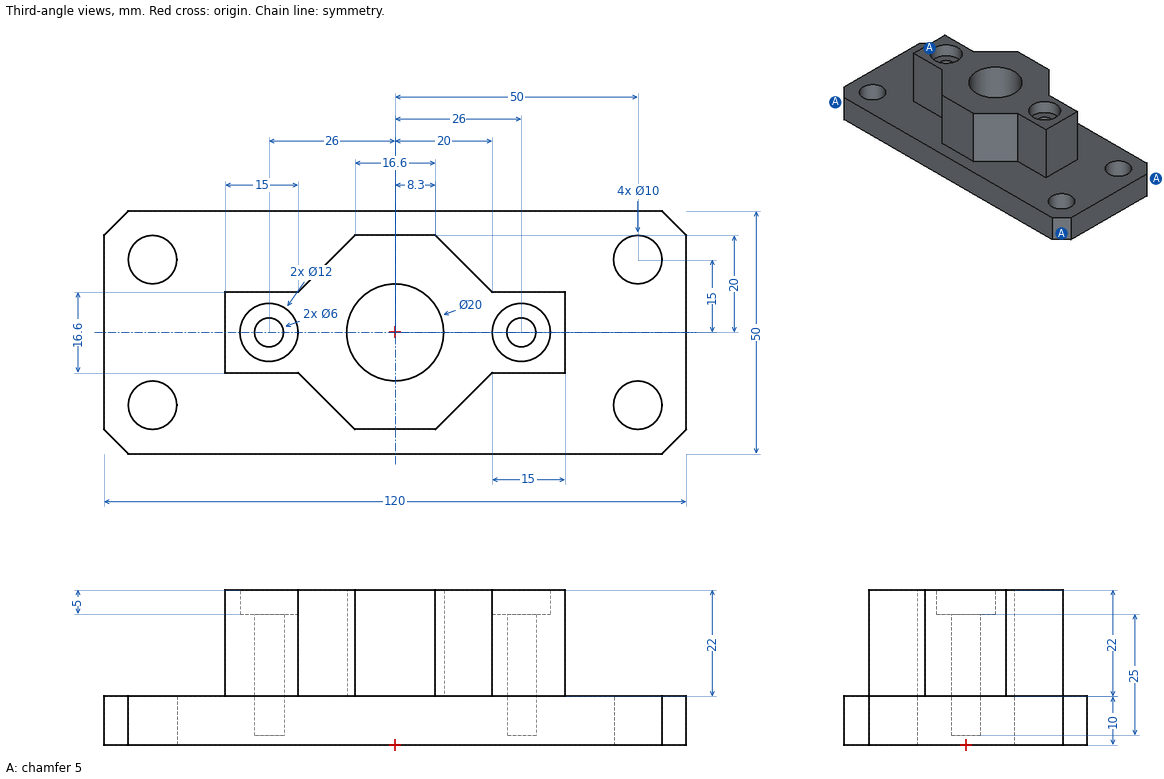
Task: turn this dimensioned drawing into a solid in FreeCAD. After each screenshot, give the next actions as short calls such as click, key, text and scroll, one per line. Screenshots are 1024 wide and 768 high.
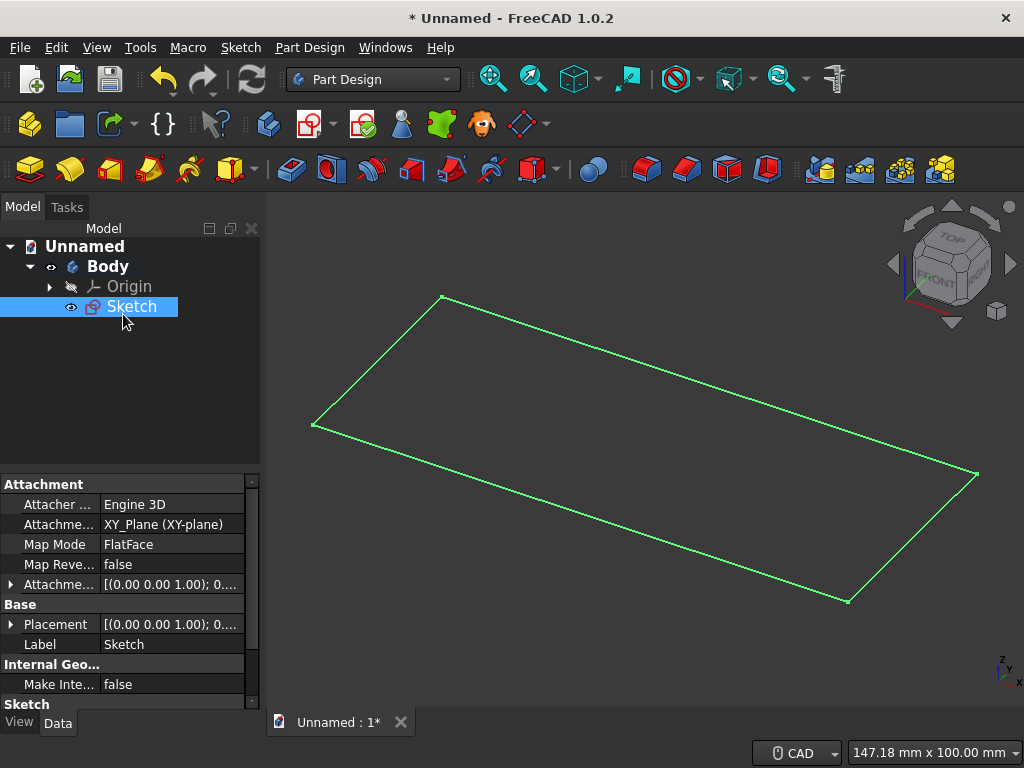
click(30, 170)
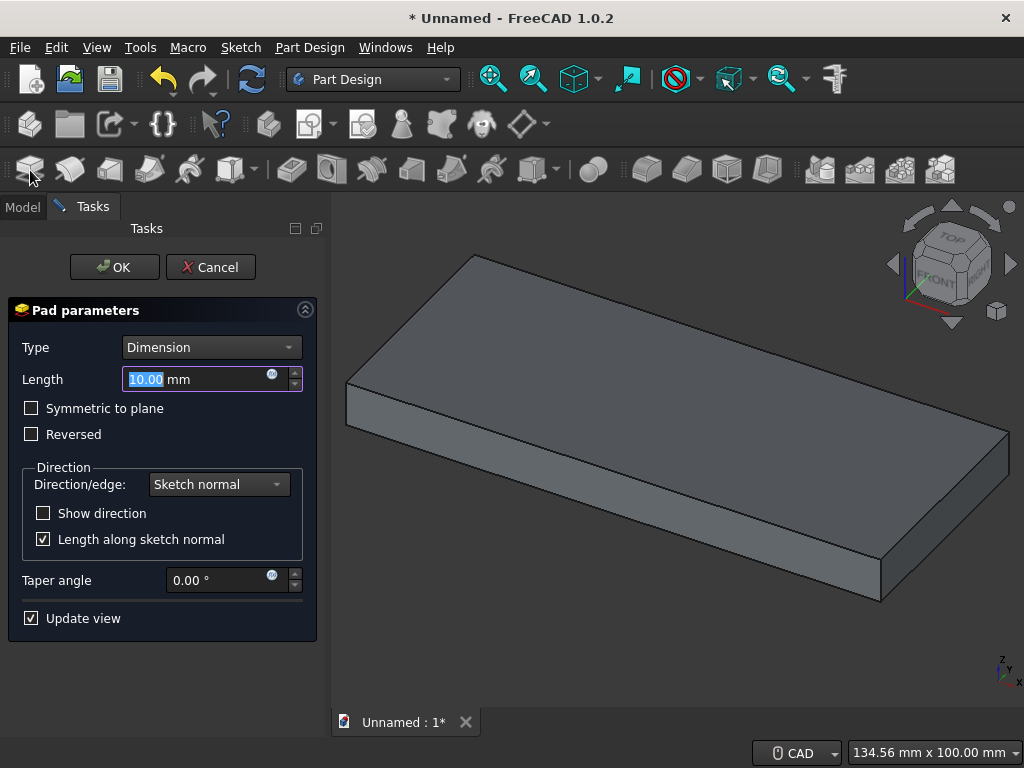
text(10)
key(Tab)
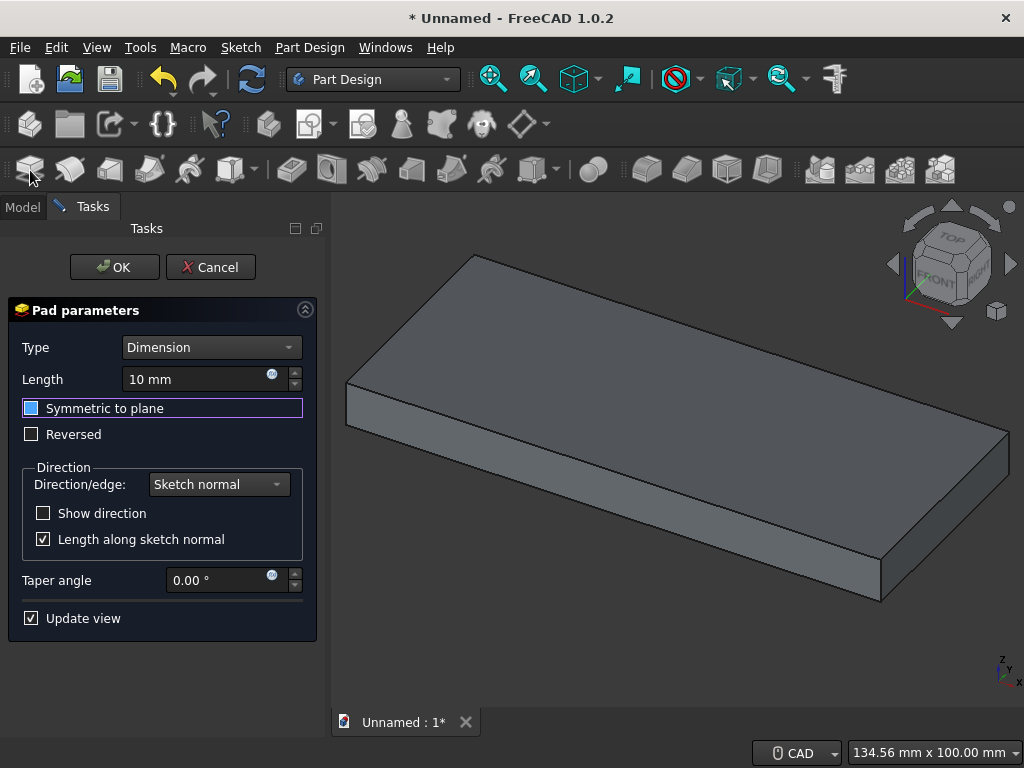
click(115, 267)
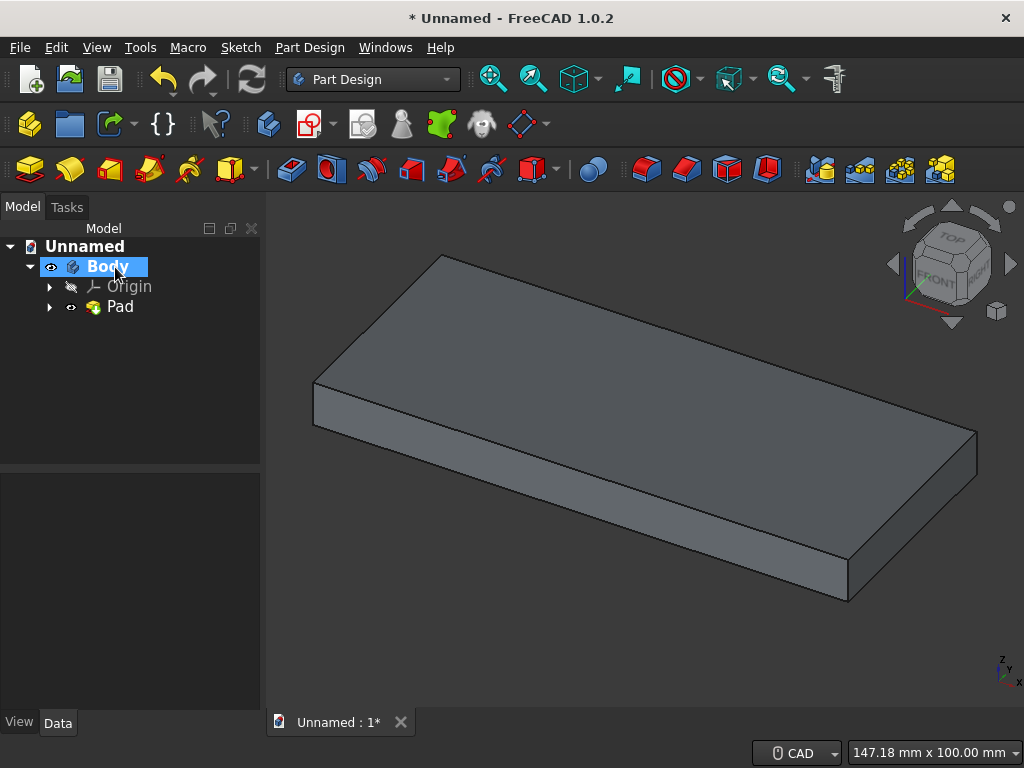
click(798, 457)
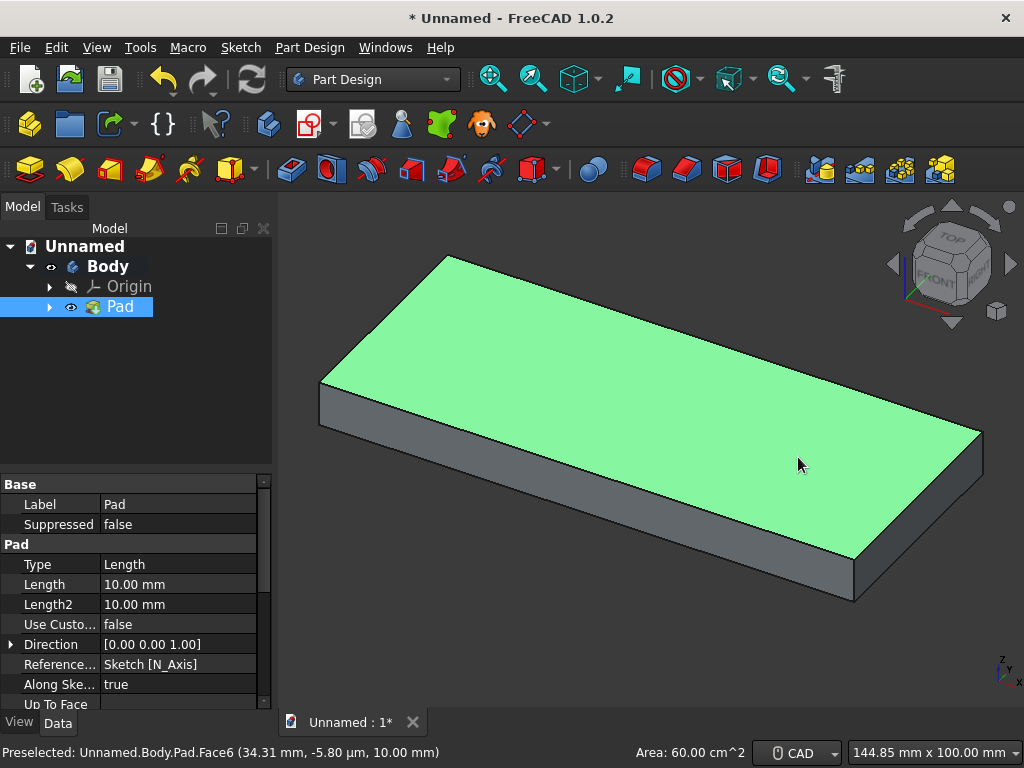
click(310, 124)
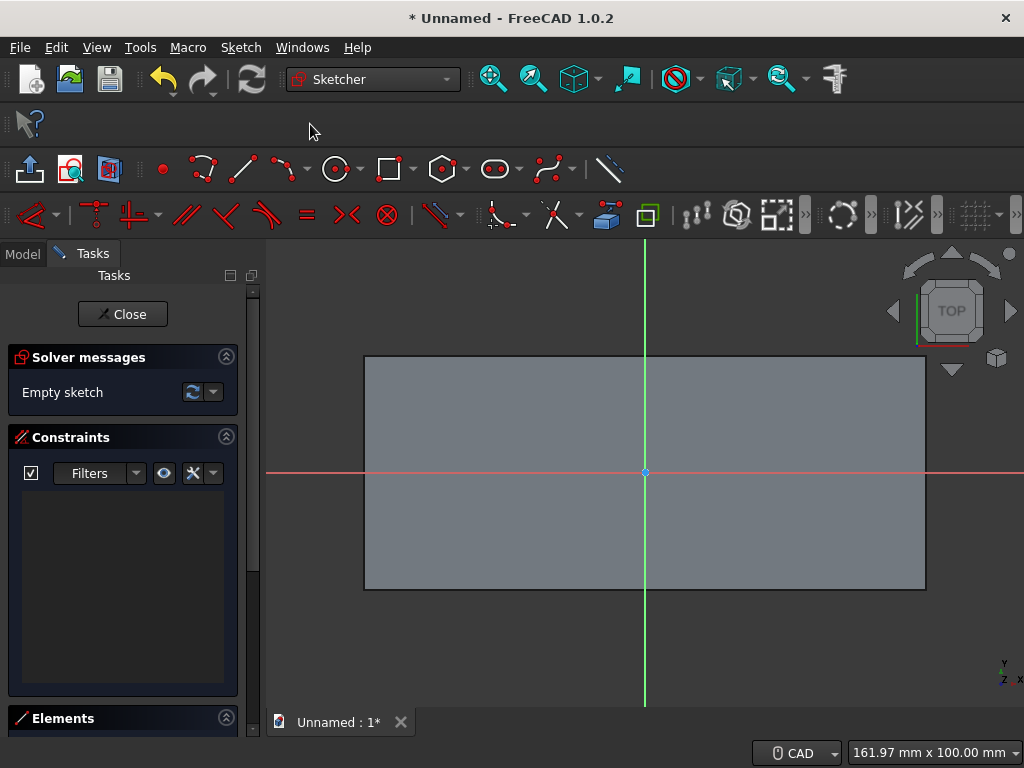
click(204, 170)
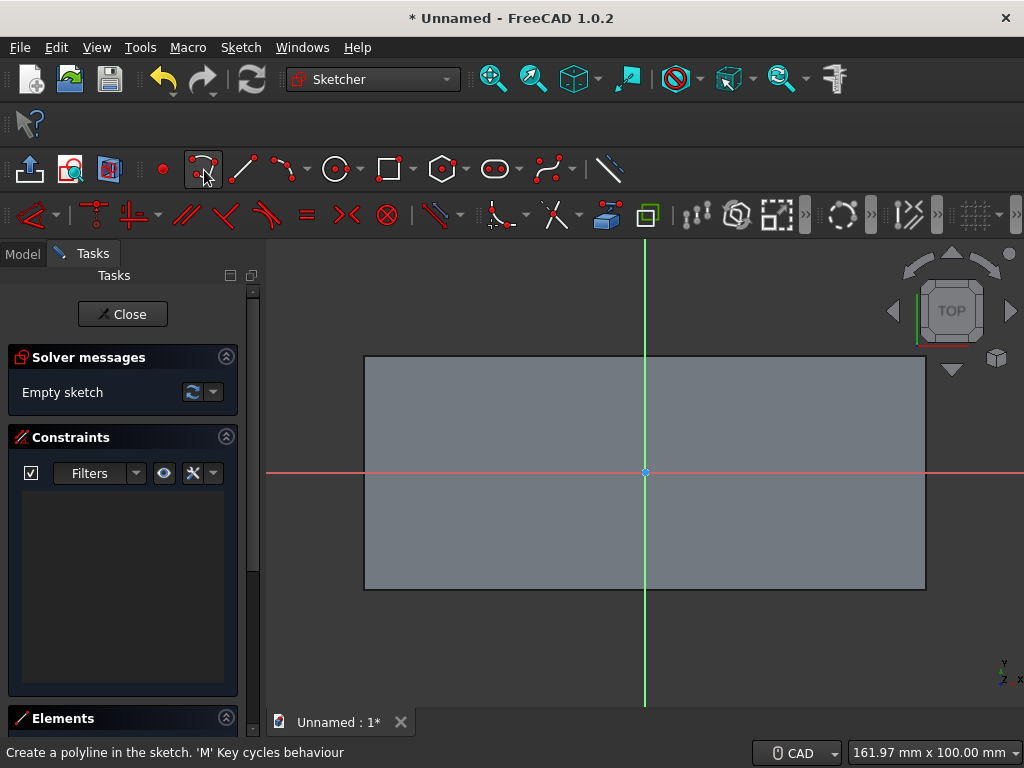
click(739, 434)
click(684, 379)
click(606, 379)
click(551, 434)
click(481, 434)
click(481, 512)
click(551, 512)
click(606, 567)
click(684, 567)
click(739, 512)
click(809, 512)
click(809, 434)
click(739, 435)
key(Escape)
key(Escape)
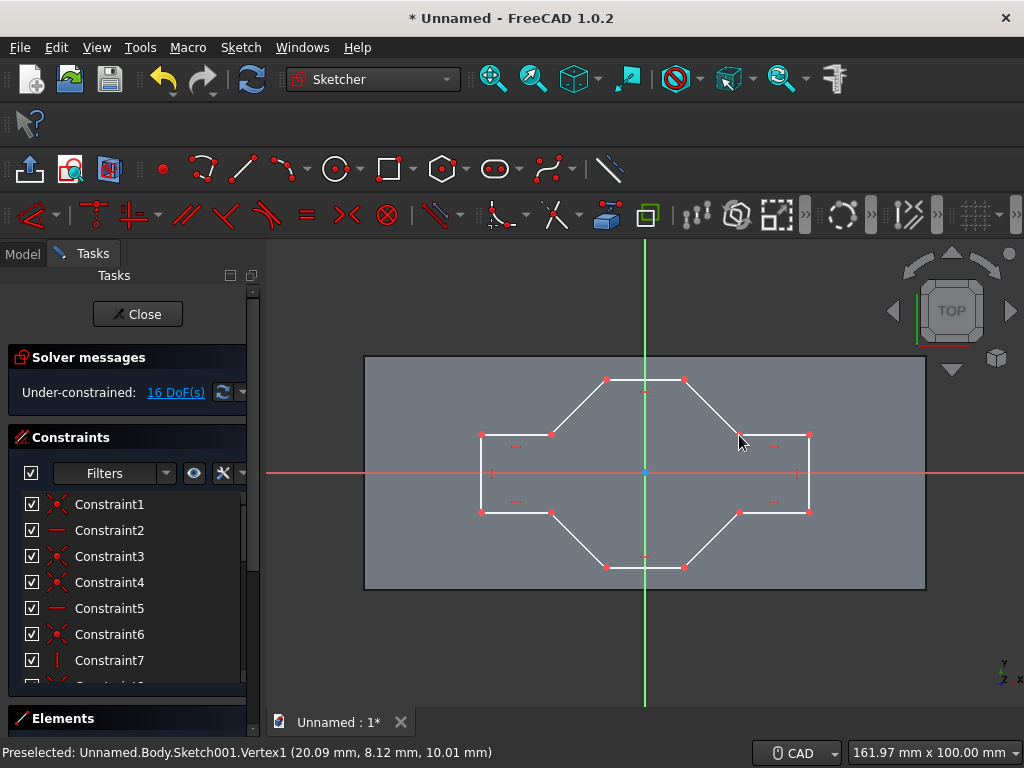
click(739, 435)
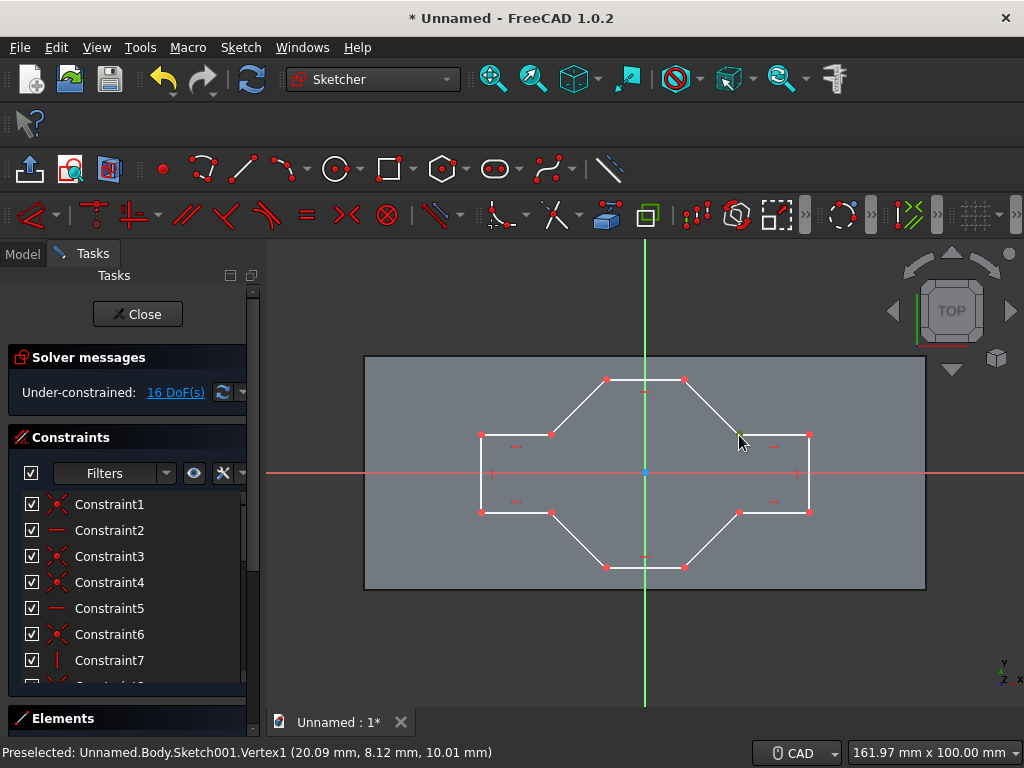
click(551, 435)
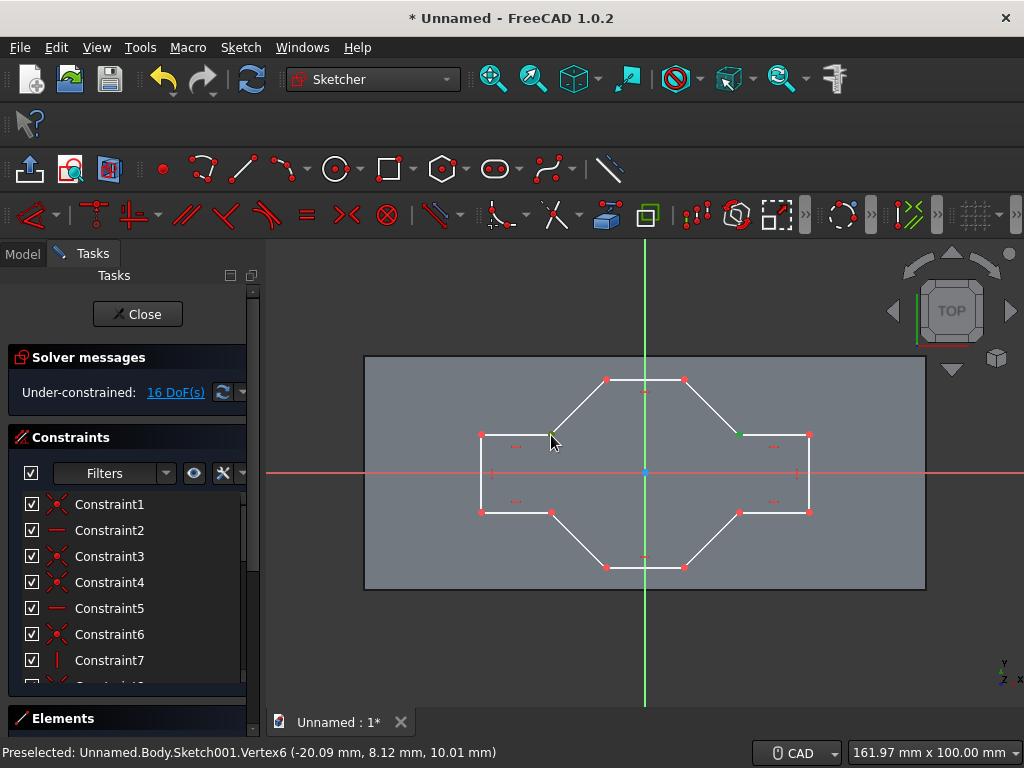
click(645, 650)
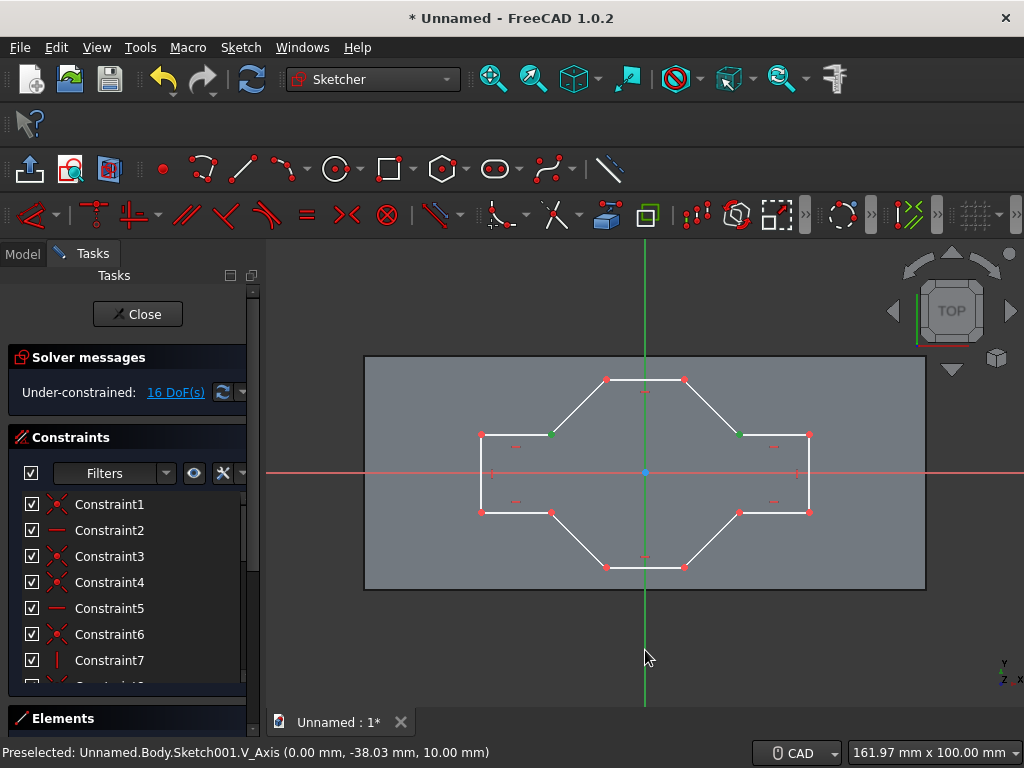
click(348, 216)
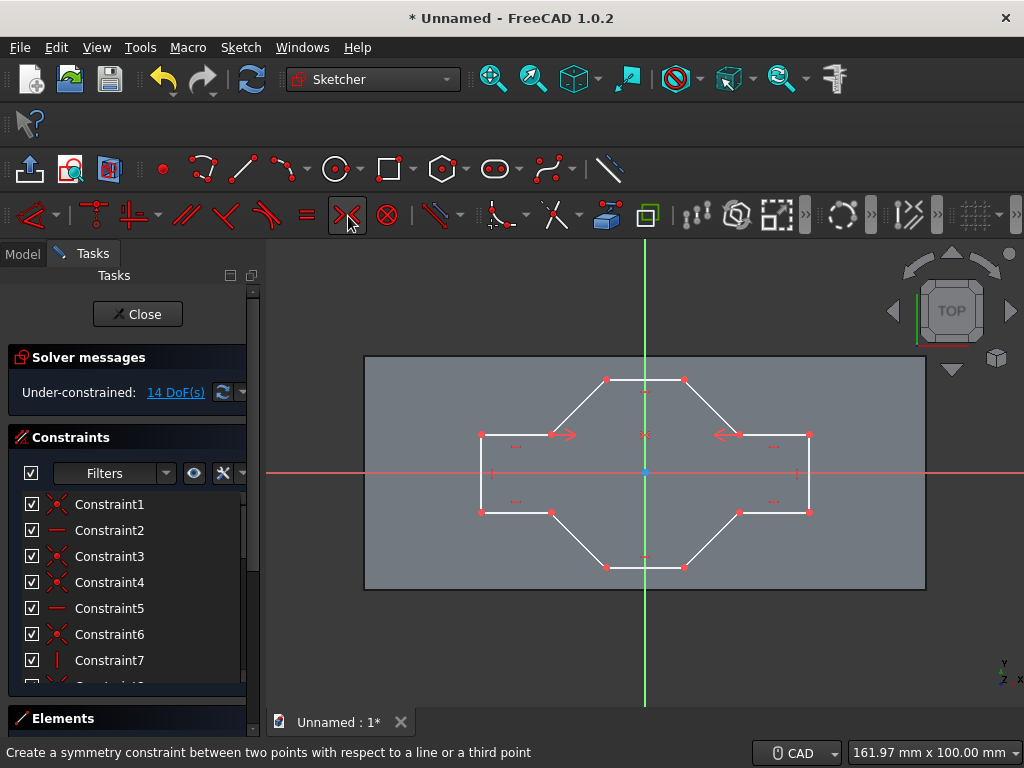
click(551, 435)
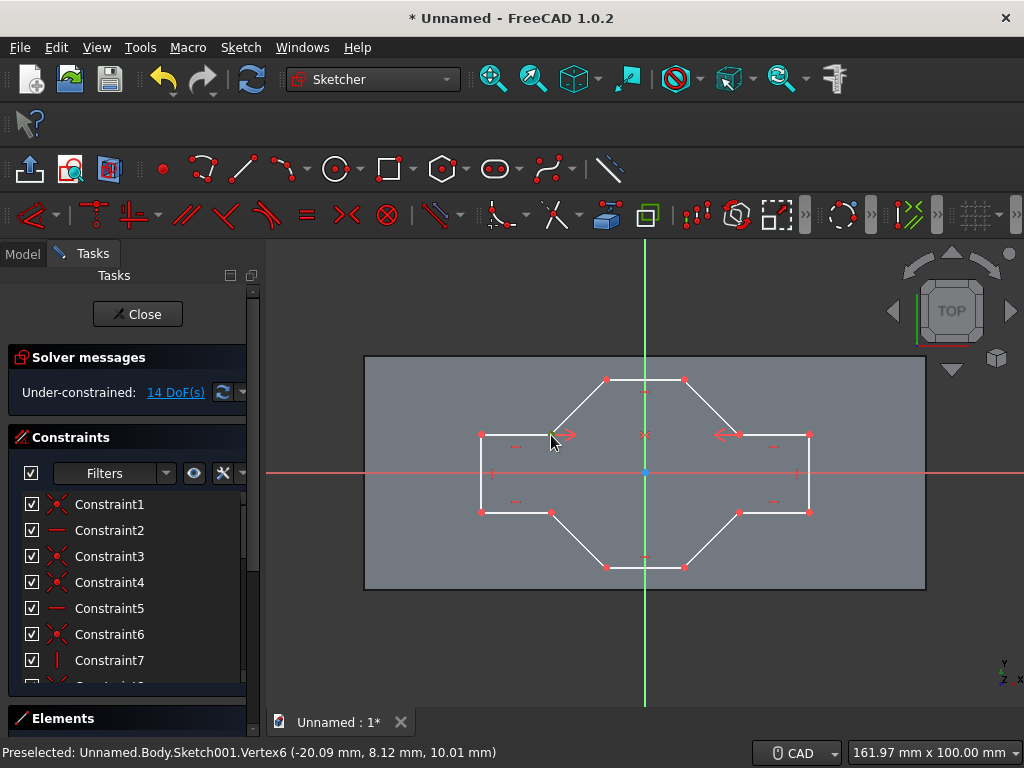
click(551, 513)